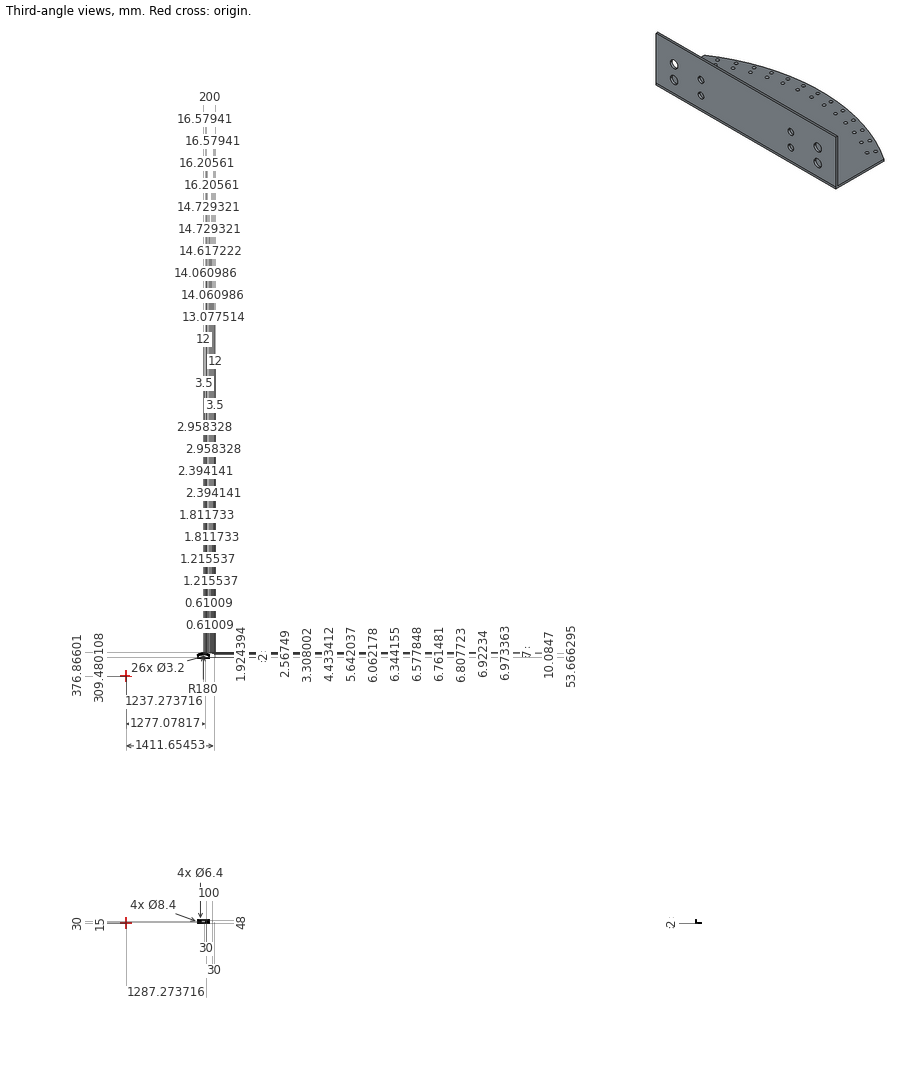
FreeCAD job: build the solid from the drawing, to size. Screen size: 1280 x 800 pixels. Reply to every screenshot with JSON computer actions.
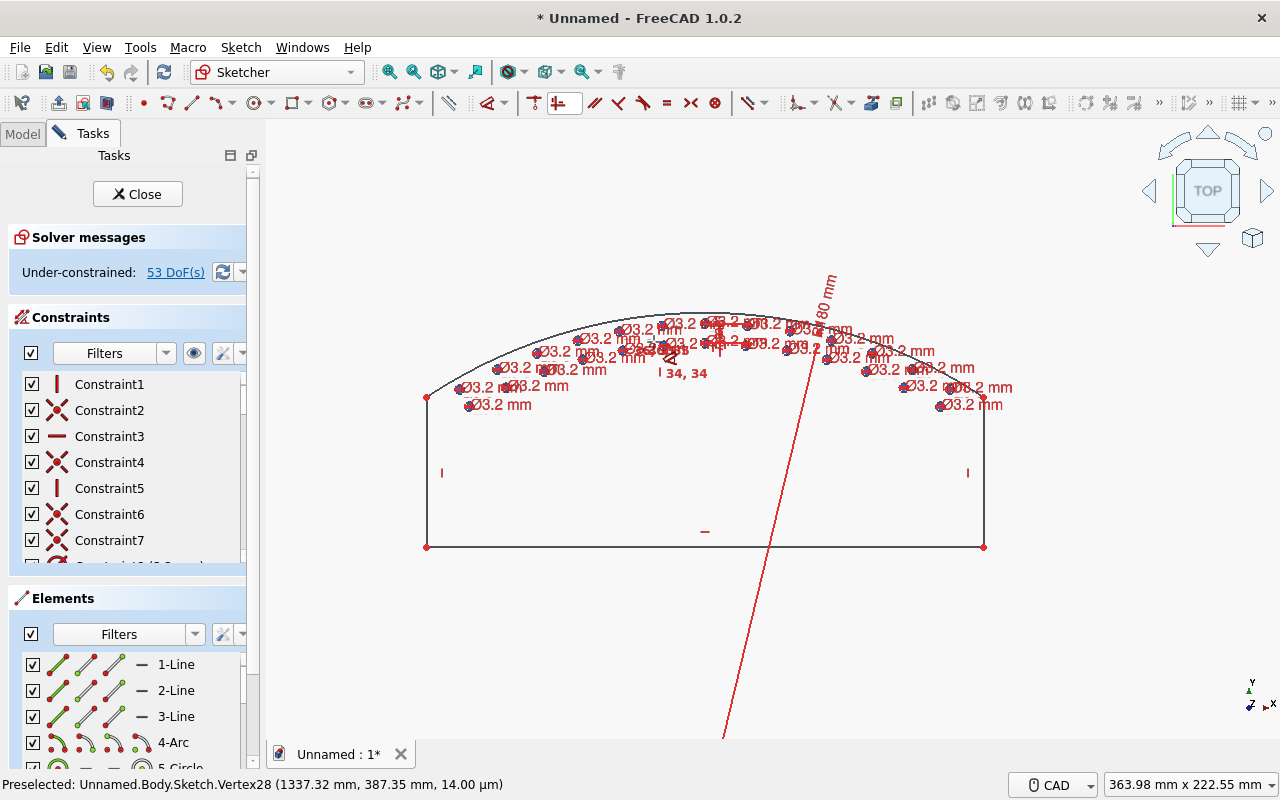
{"action": "left_click", "coordinate": [594, 547]}
{"action": "left_click", "coordinate": [705, 581]}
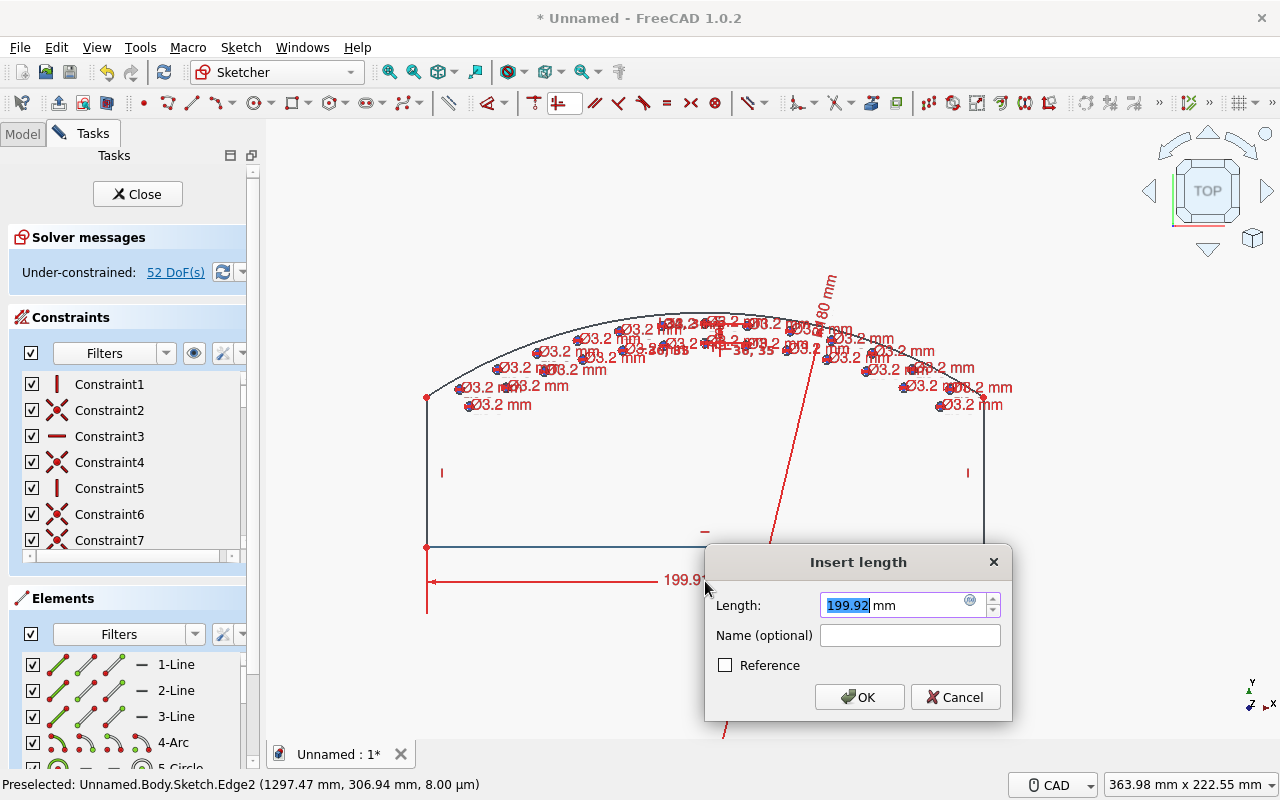
{"action": "type", "text": "200"}
{"action": "key", "text": "Return"}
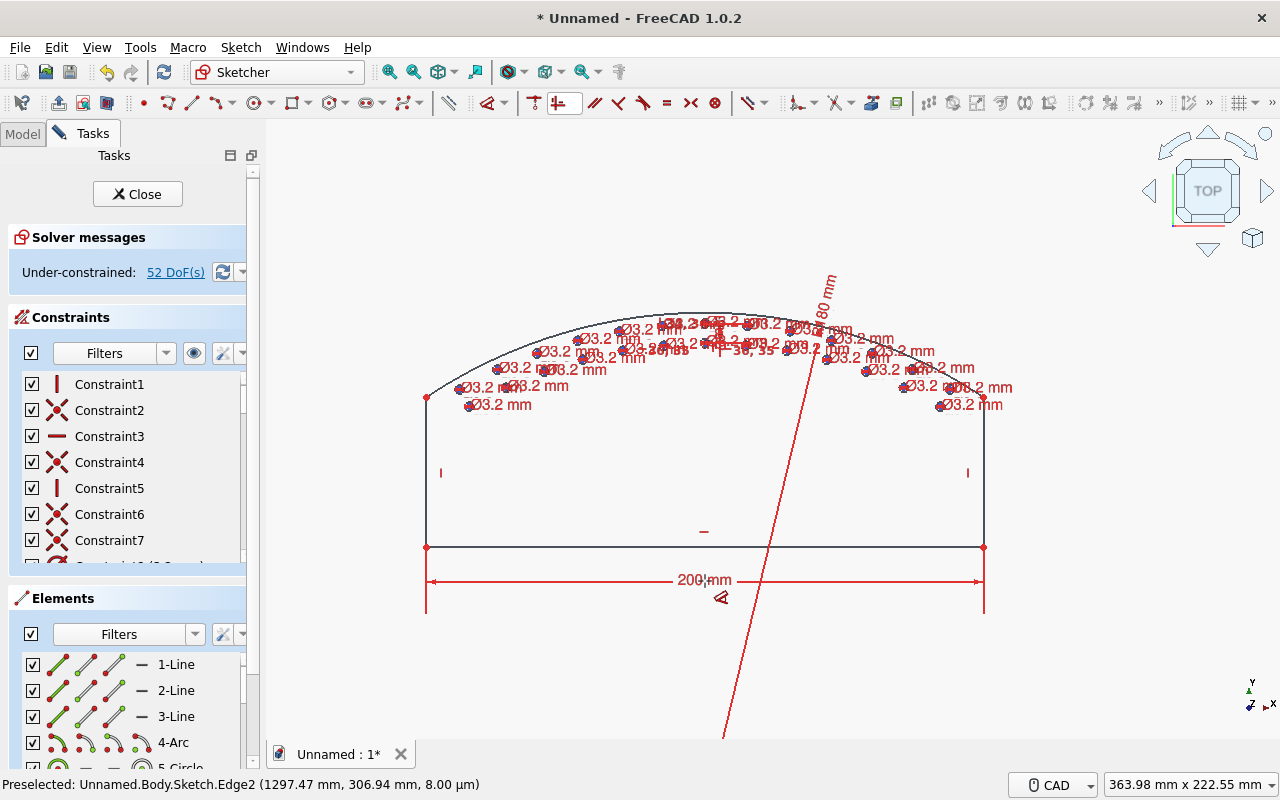
{"action": "left_click", "coordinate": [984, 397]}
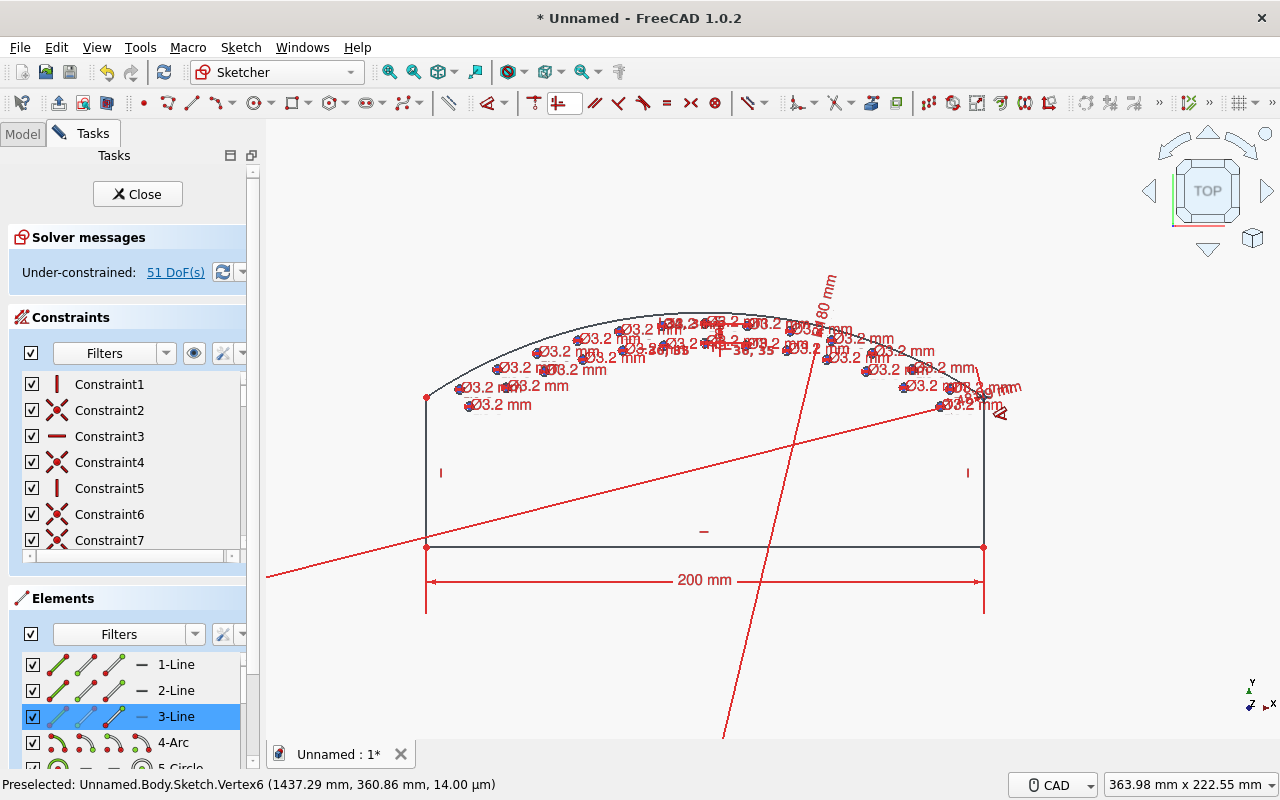
{"action": "left_click", "coordinate": [950, 390]}
{"action": "left_click", "coordinate": [967, 356]}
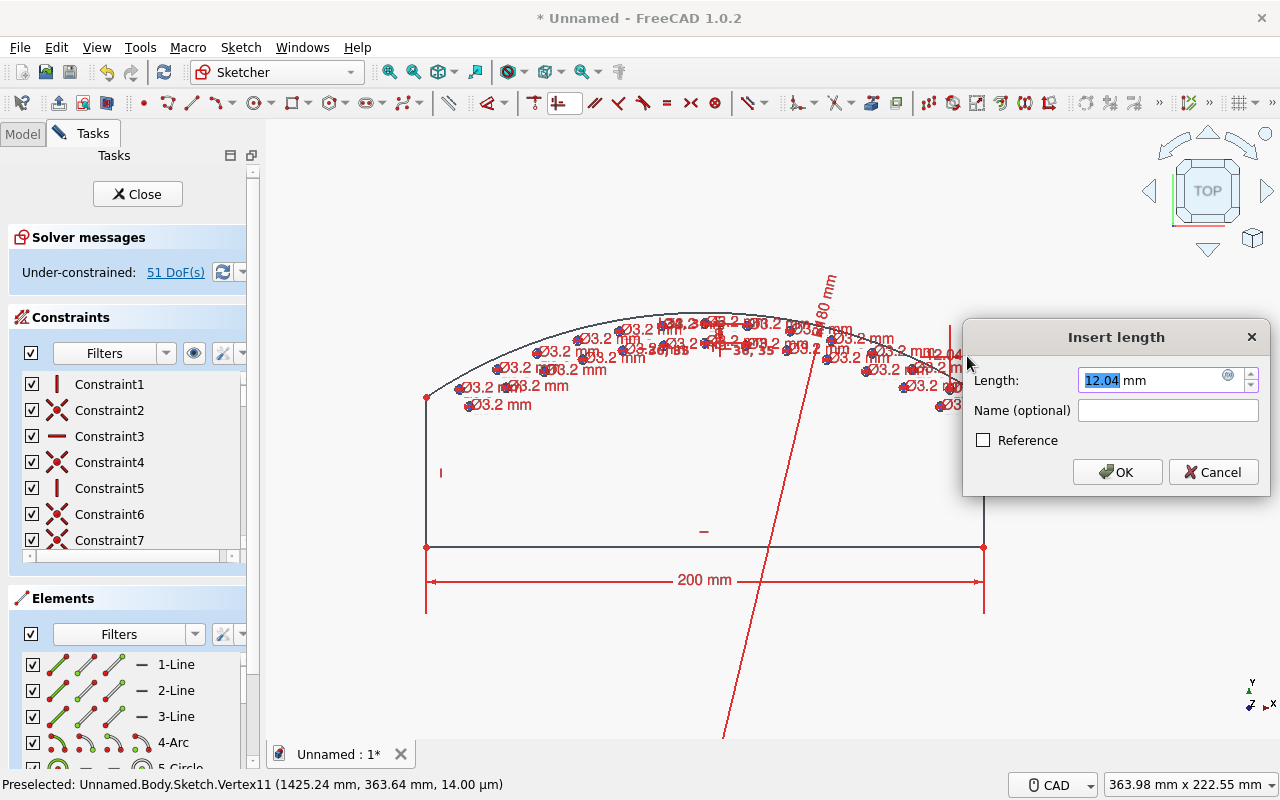
{"action": "type", "text": "12"}
{"action": "key", "text": "Return"}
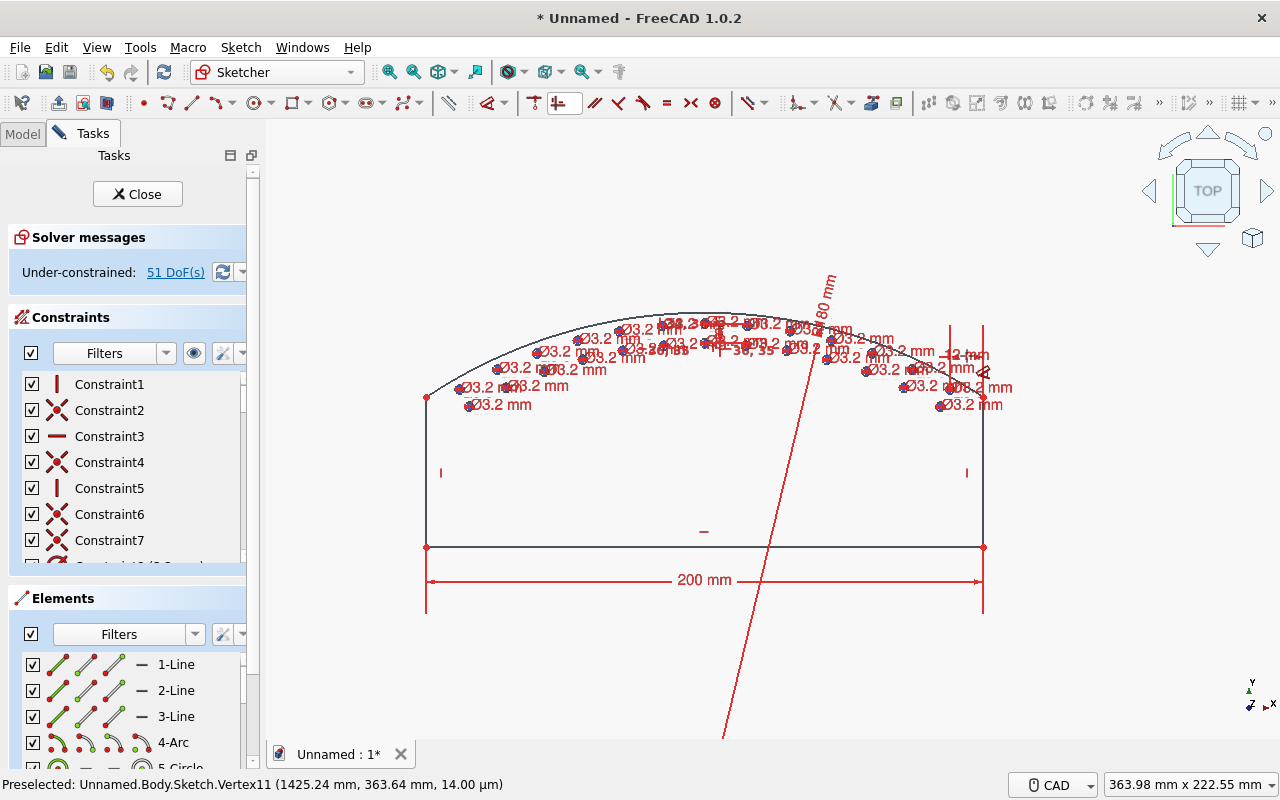
{"action": "left_click", "coordinate": [426, 397]}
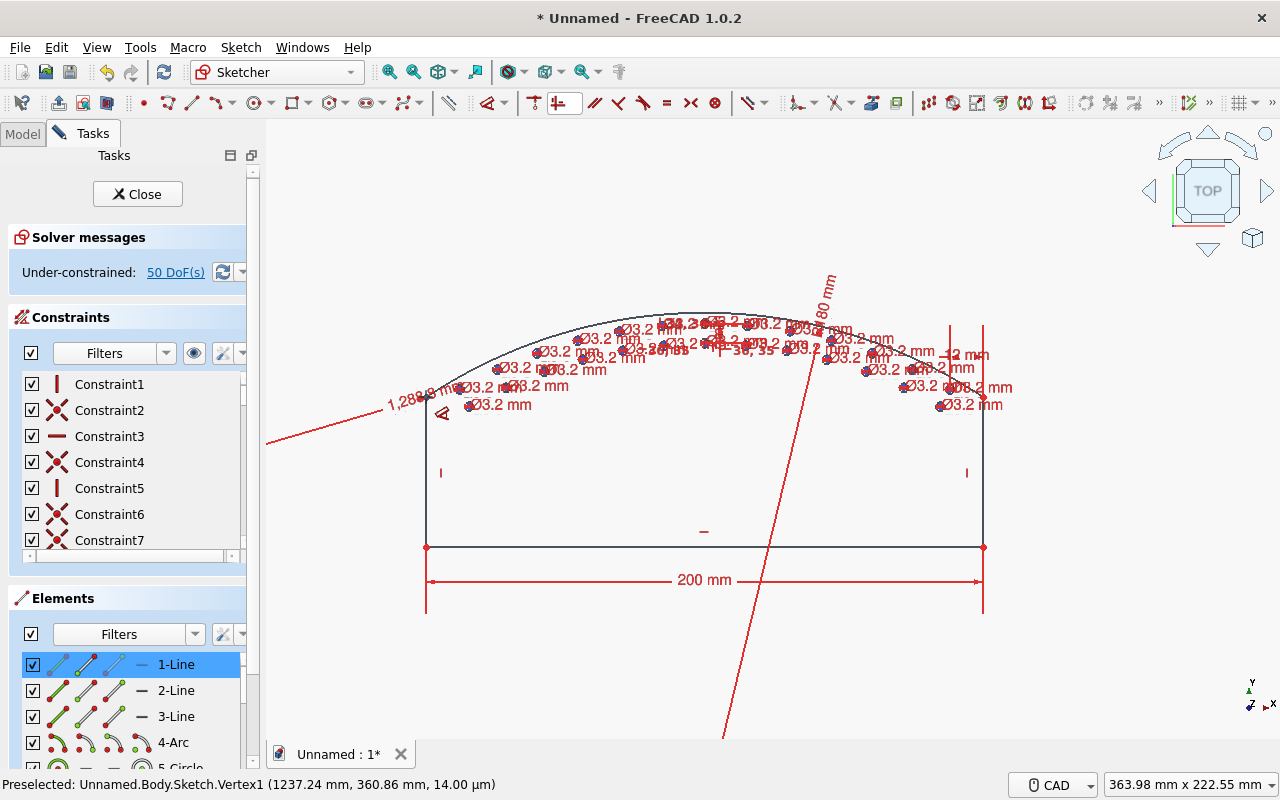
{"action": "left_click", "coordinate": [460, 390]}
{"action": "left_click", "coordinate": [443, 356]}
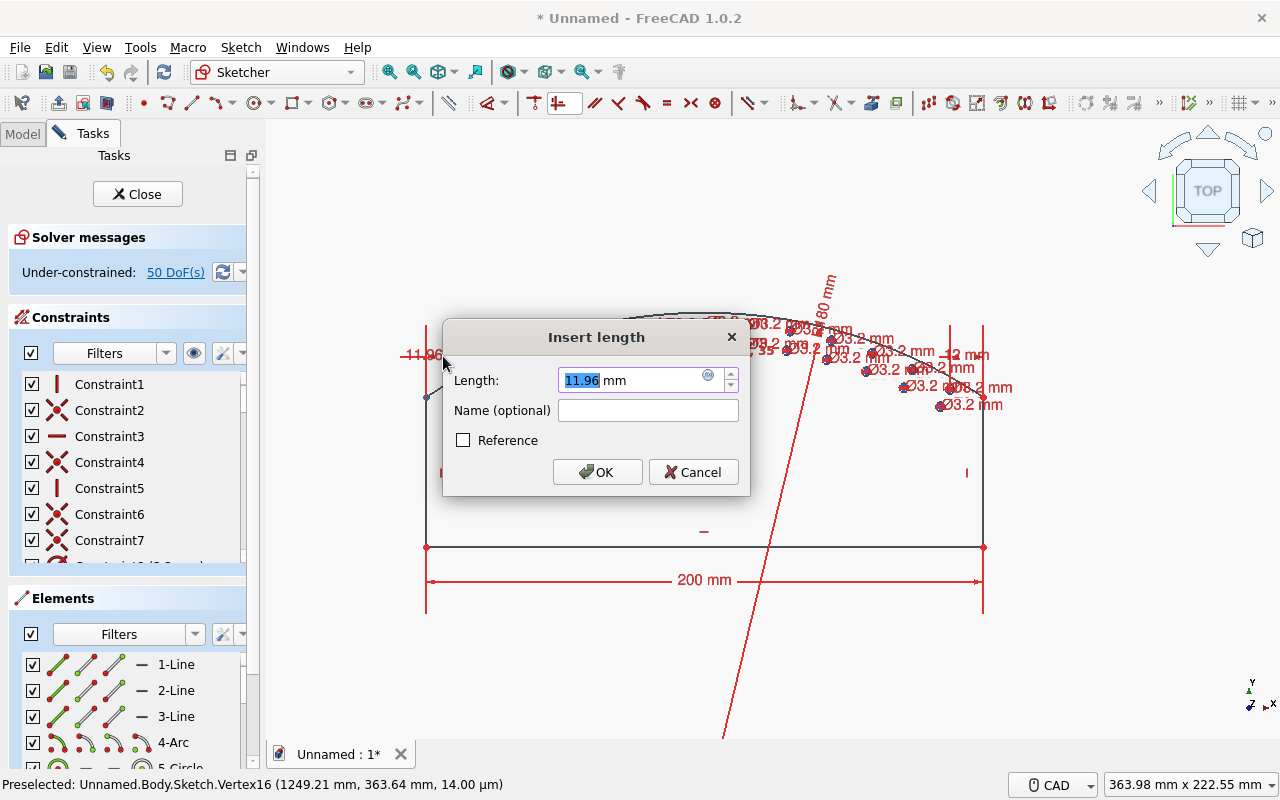
{"action": "type", "text": "12"}
{"action": "key", "text": "Return"}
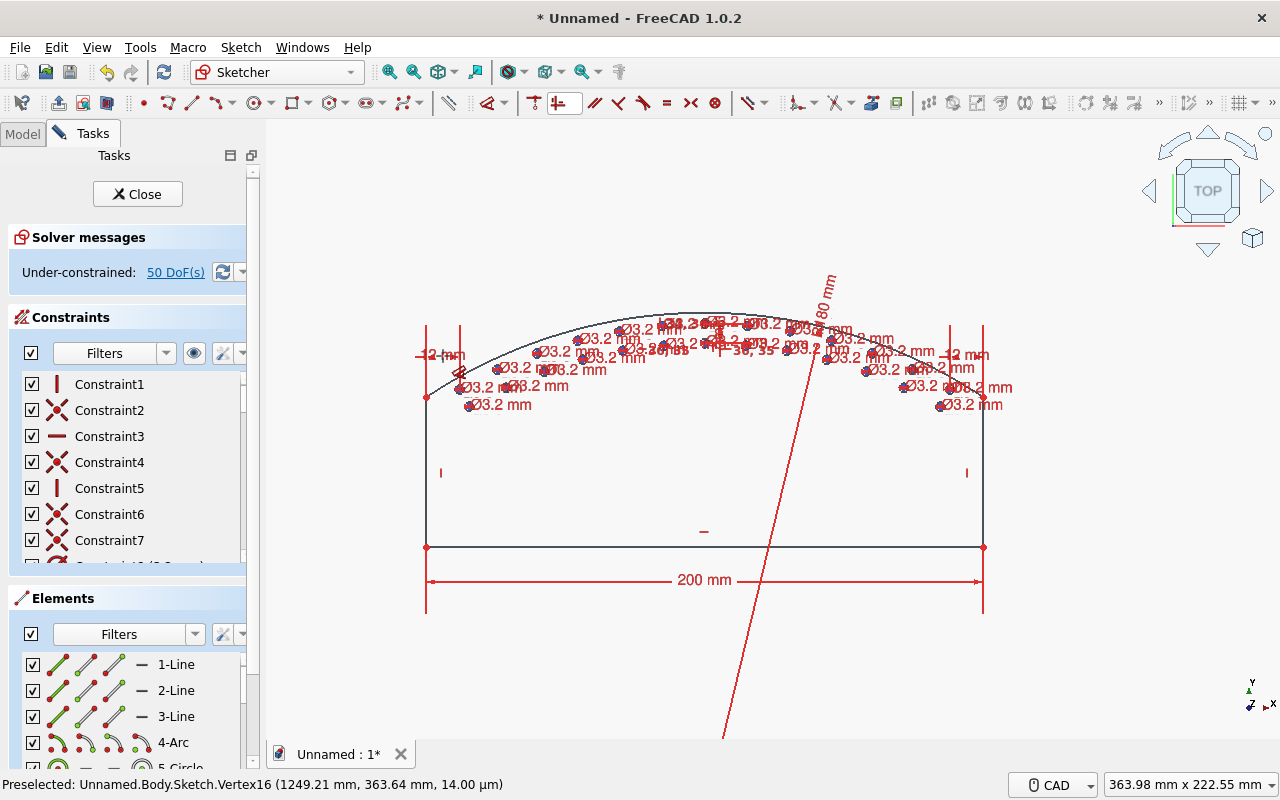
{"action": "scroll", "coordinate": [940, 407], "scroll_direction": "up", "scroll_amount": 8}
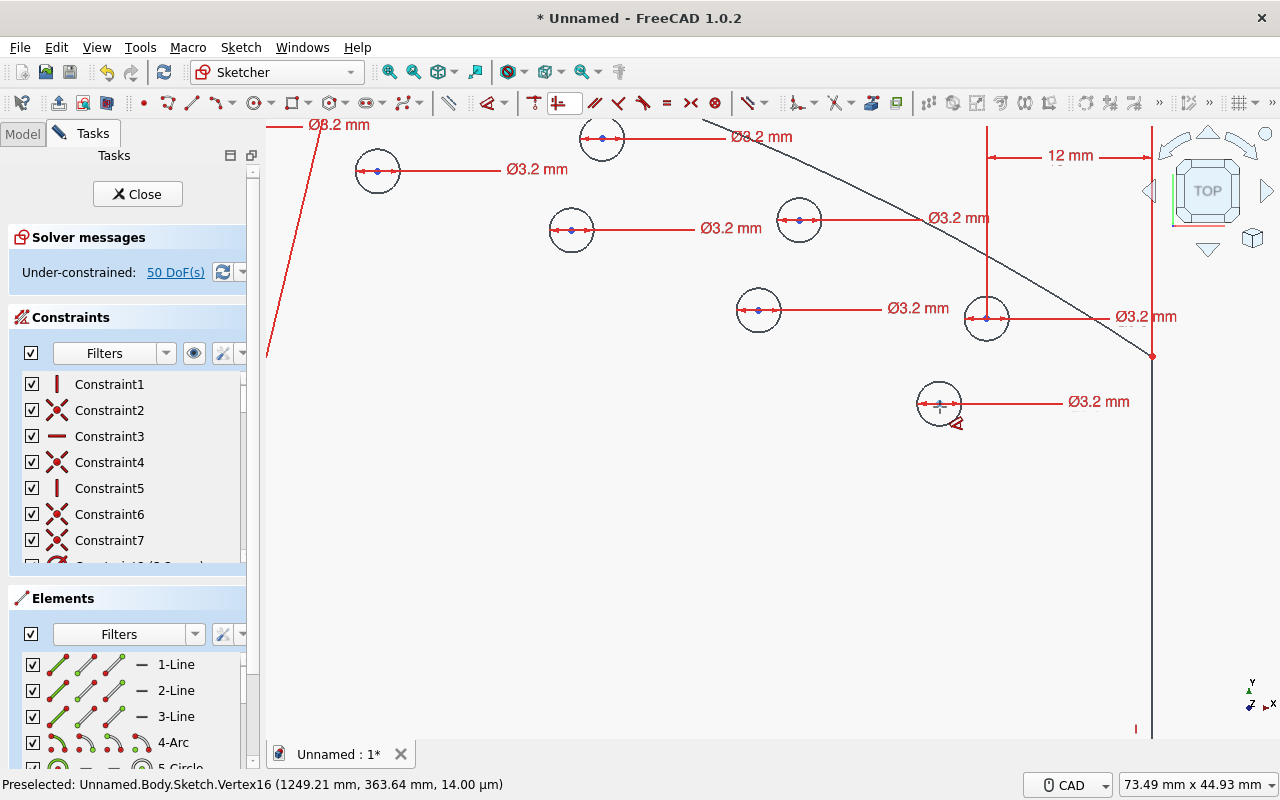
{"action": "left_click", "coordinate": [939, 404]}